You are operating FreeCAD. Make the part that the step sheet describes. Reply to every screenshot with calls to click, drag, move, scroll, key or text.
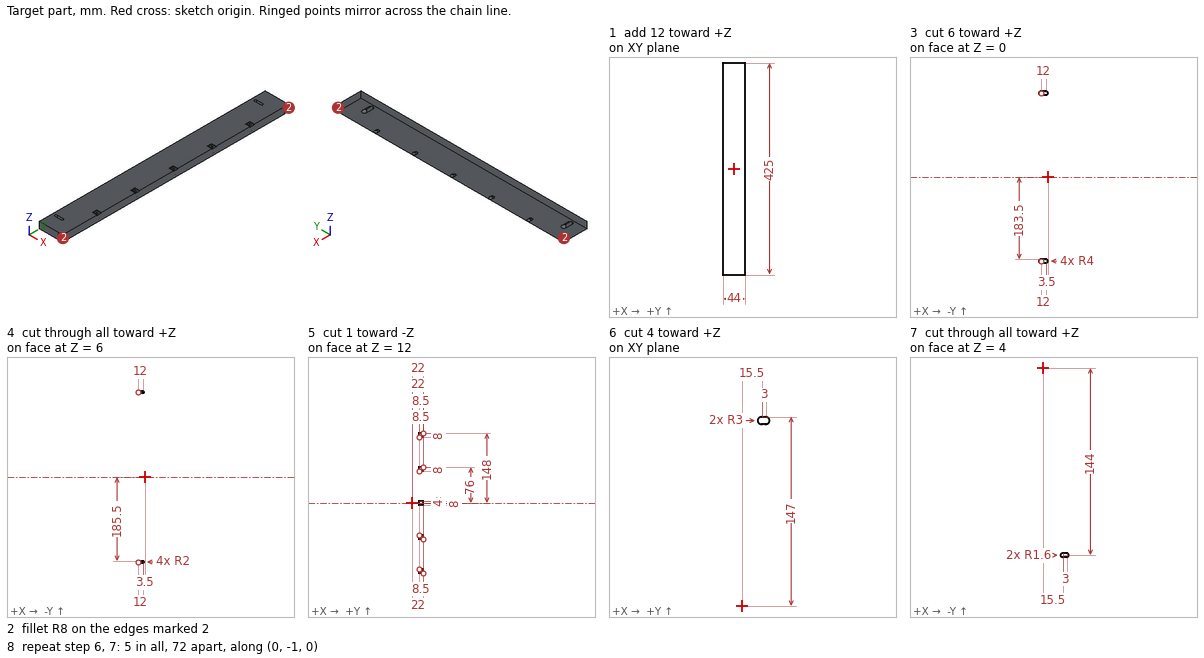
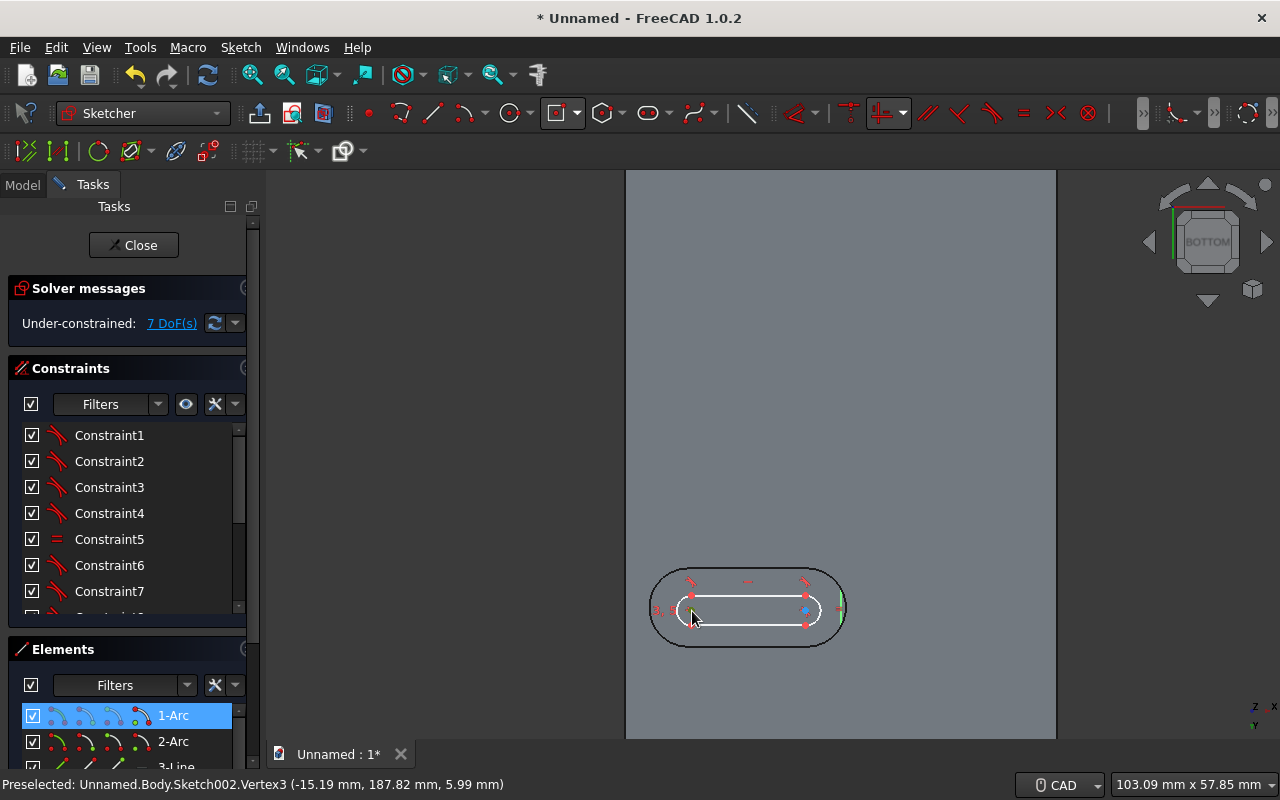
scroll(699, 623, down, 12)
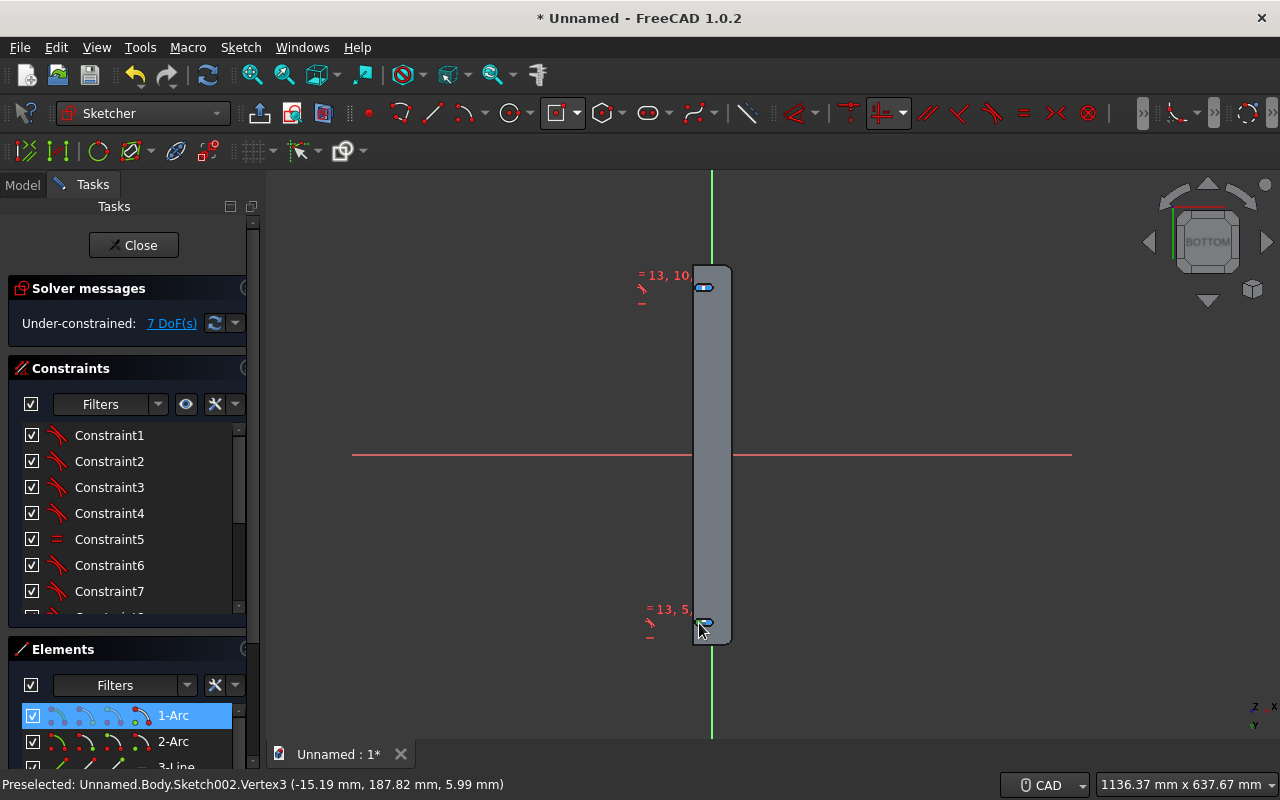
scroll(699, 288, up, 12)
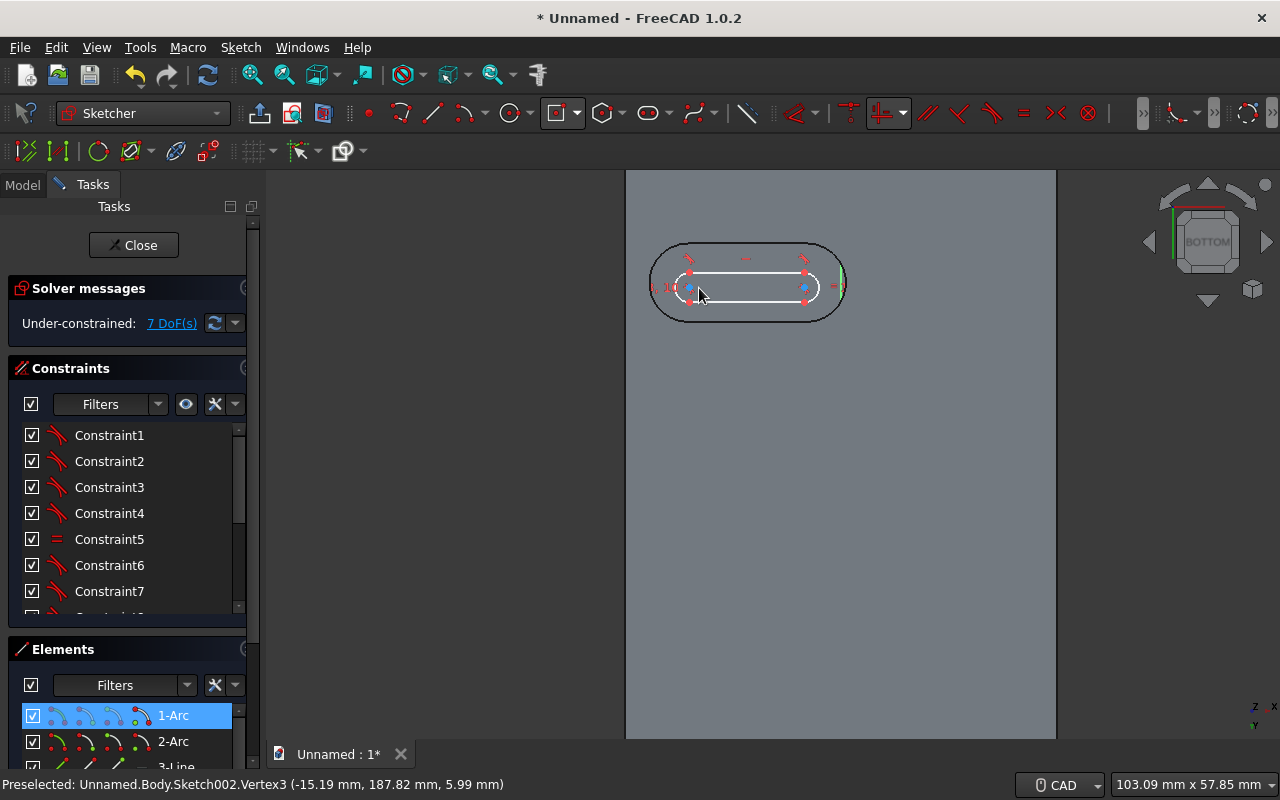
click(690, 288)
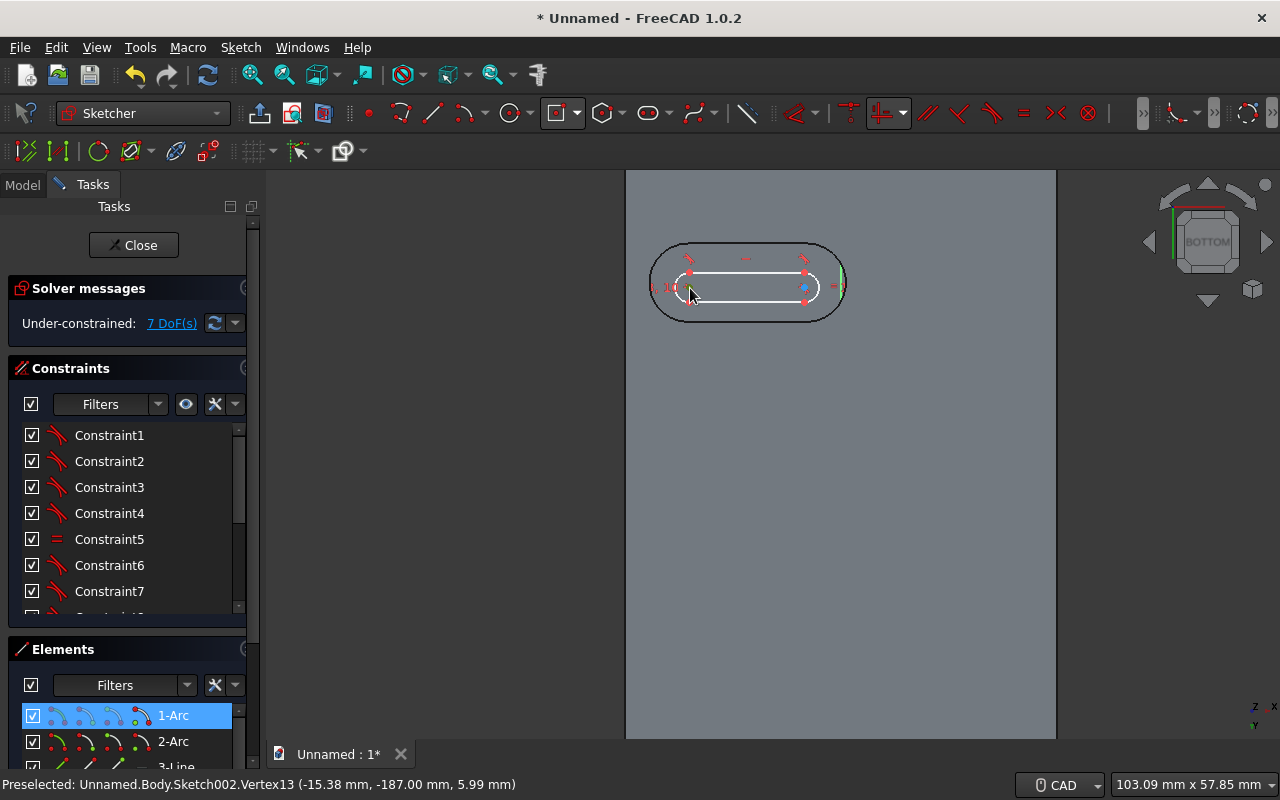
scroll(699, 288, down, 12)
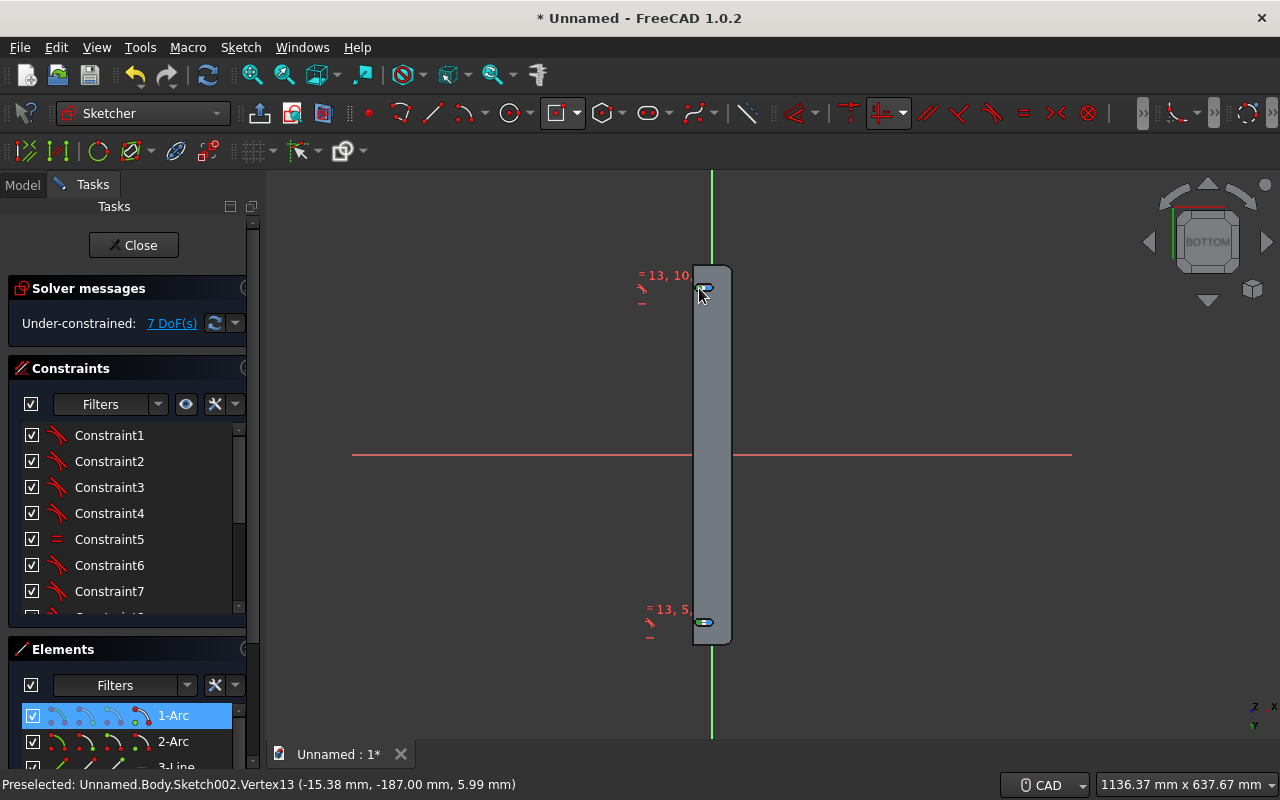
click(353, 455)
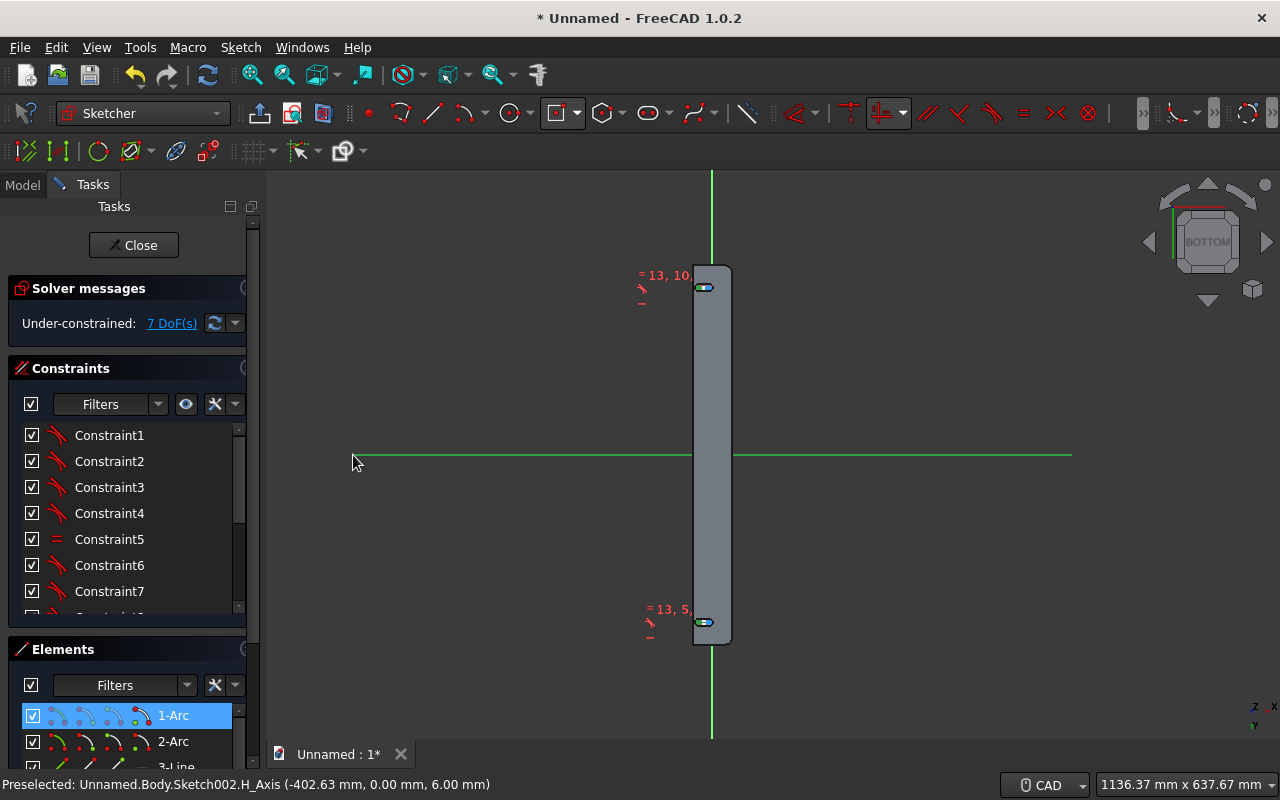
click(1056, 114)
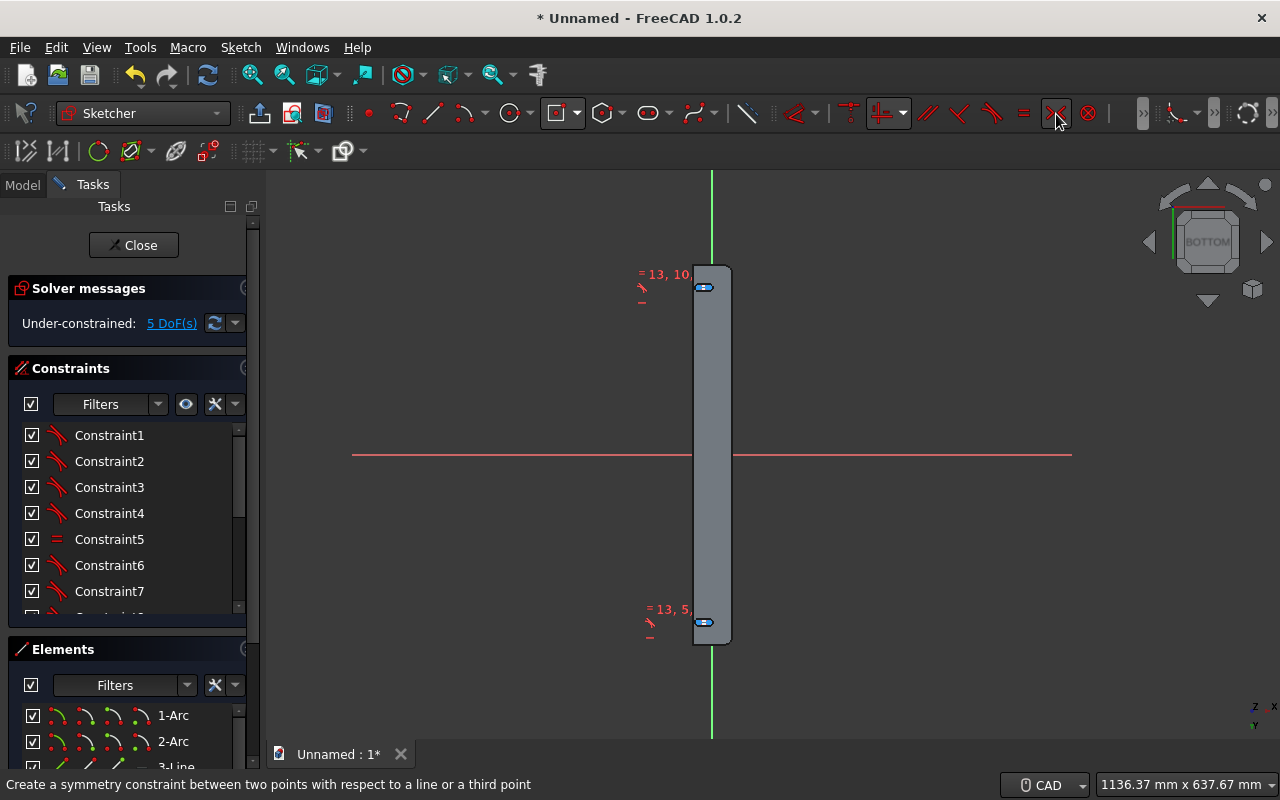
click(794, 114)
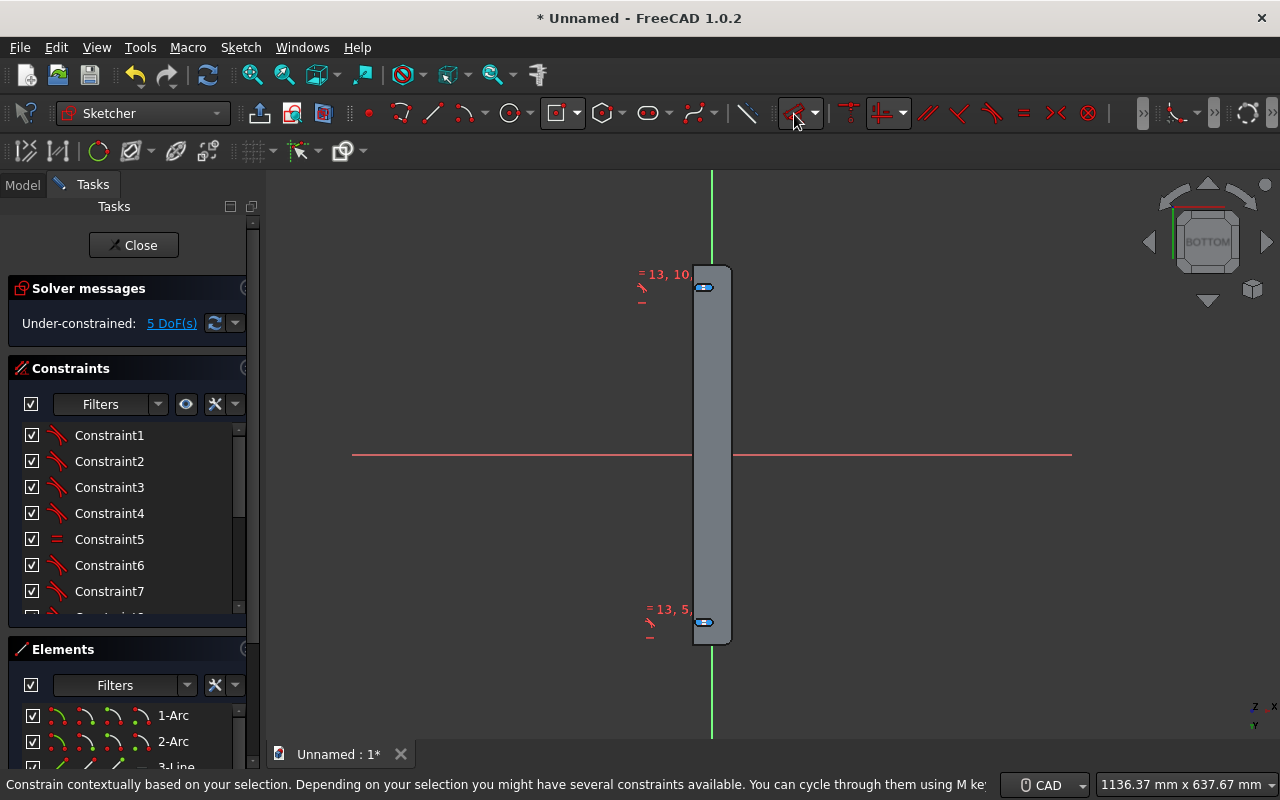
scroll(697, 622, up, 16)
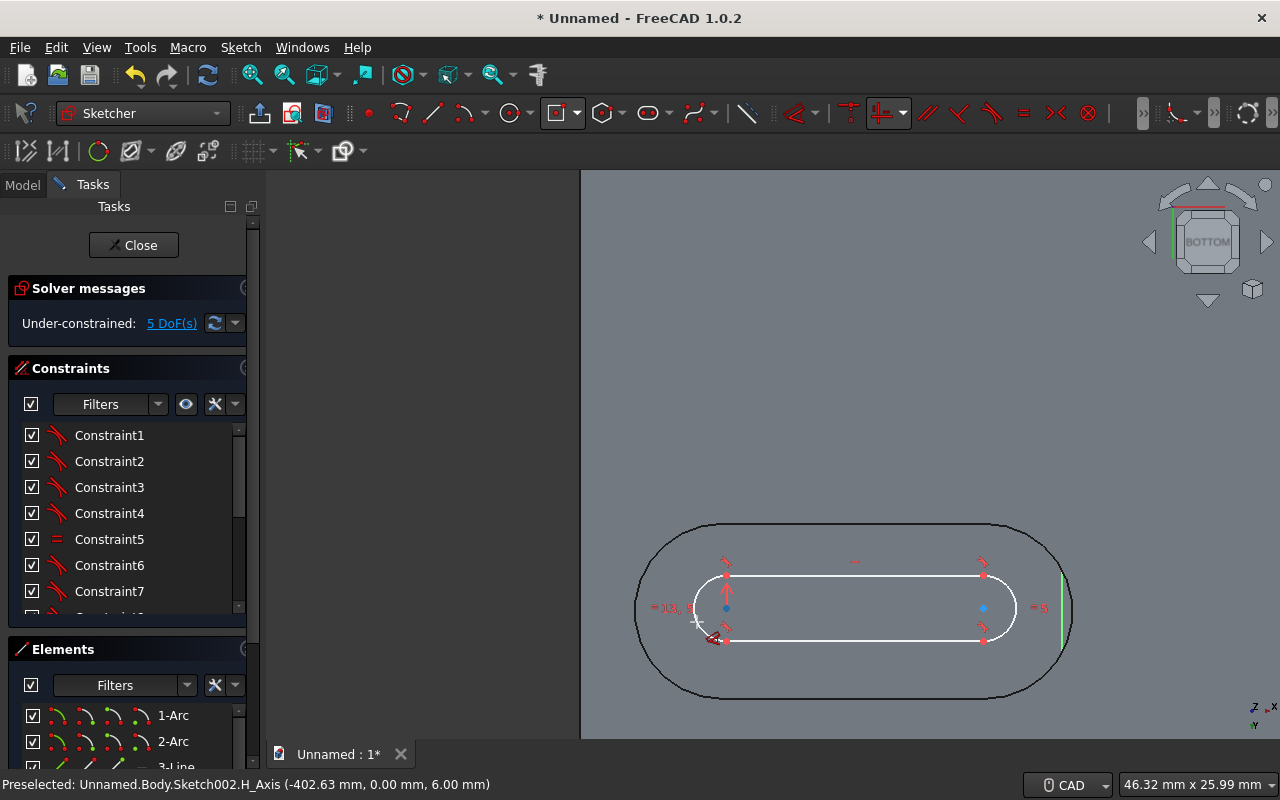
click(694, 608)
click(662, 608)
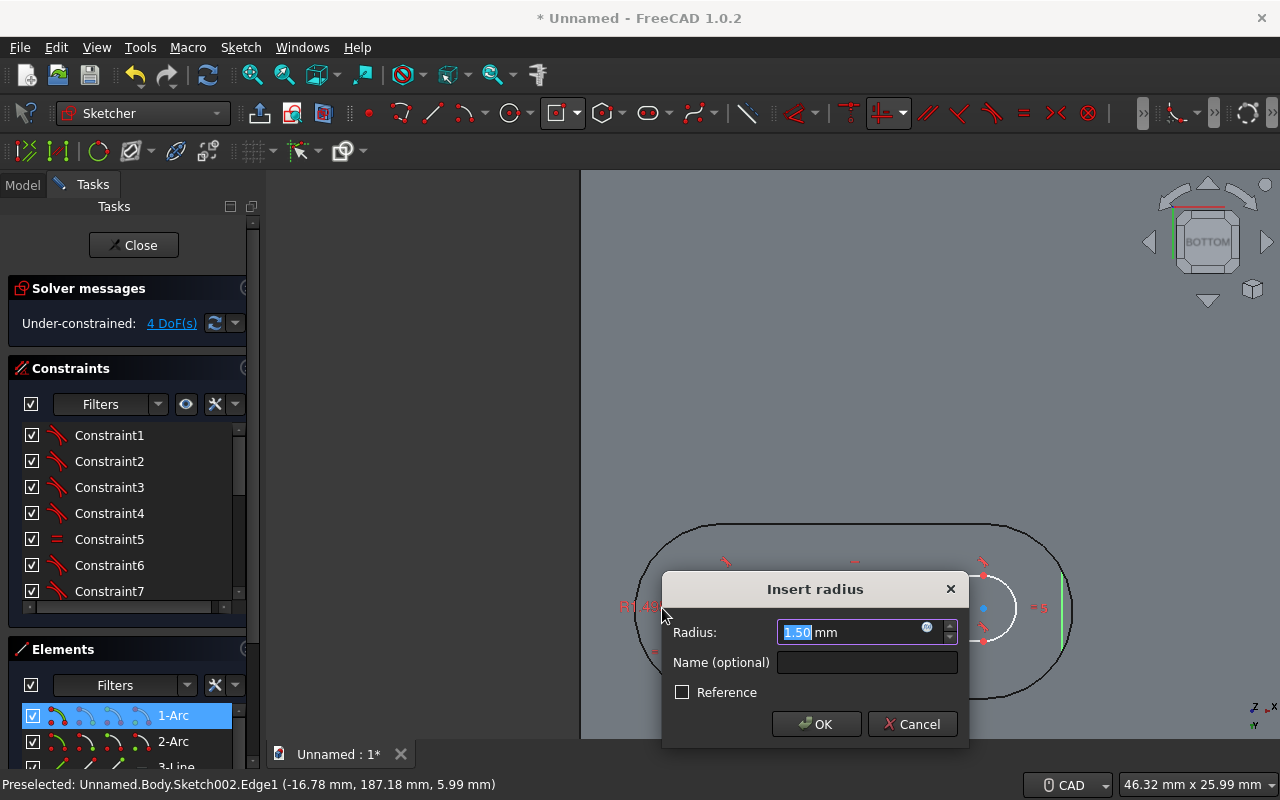
text(2)
key(Return)